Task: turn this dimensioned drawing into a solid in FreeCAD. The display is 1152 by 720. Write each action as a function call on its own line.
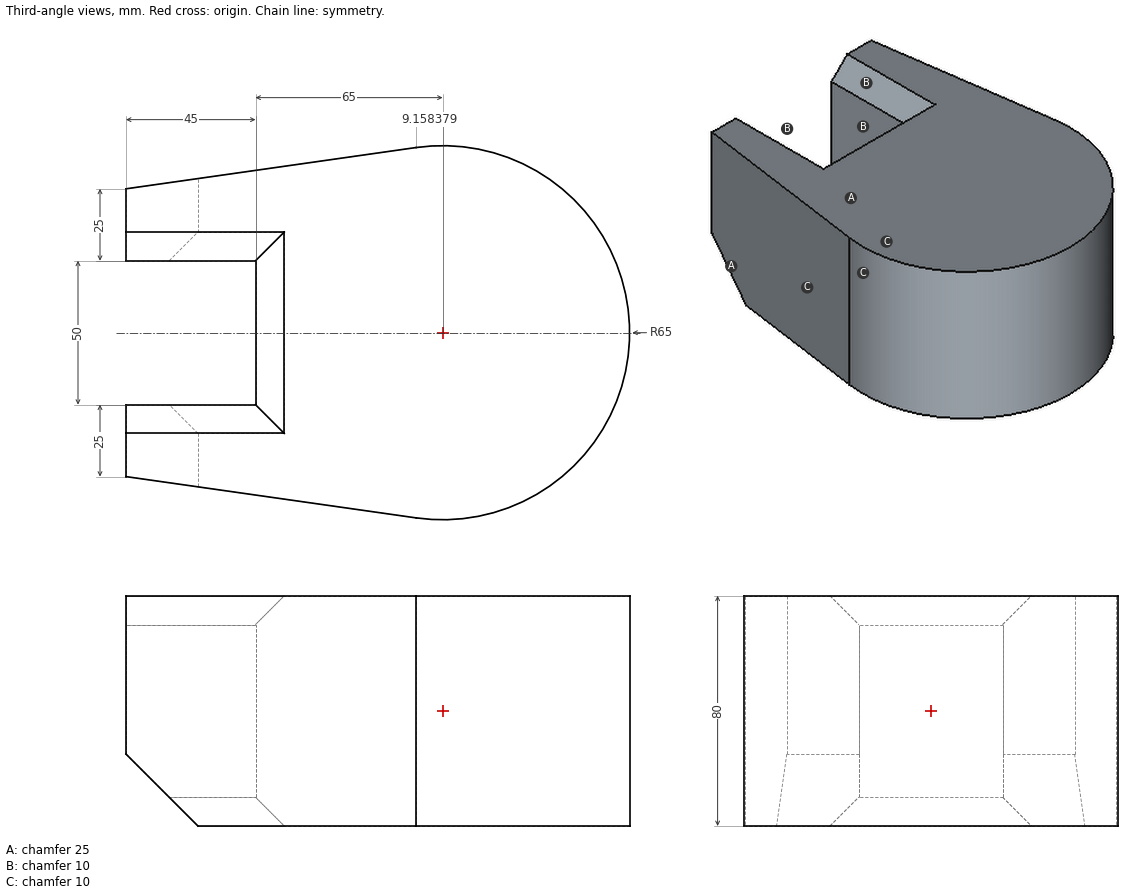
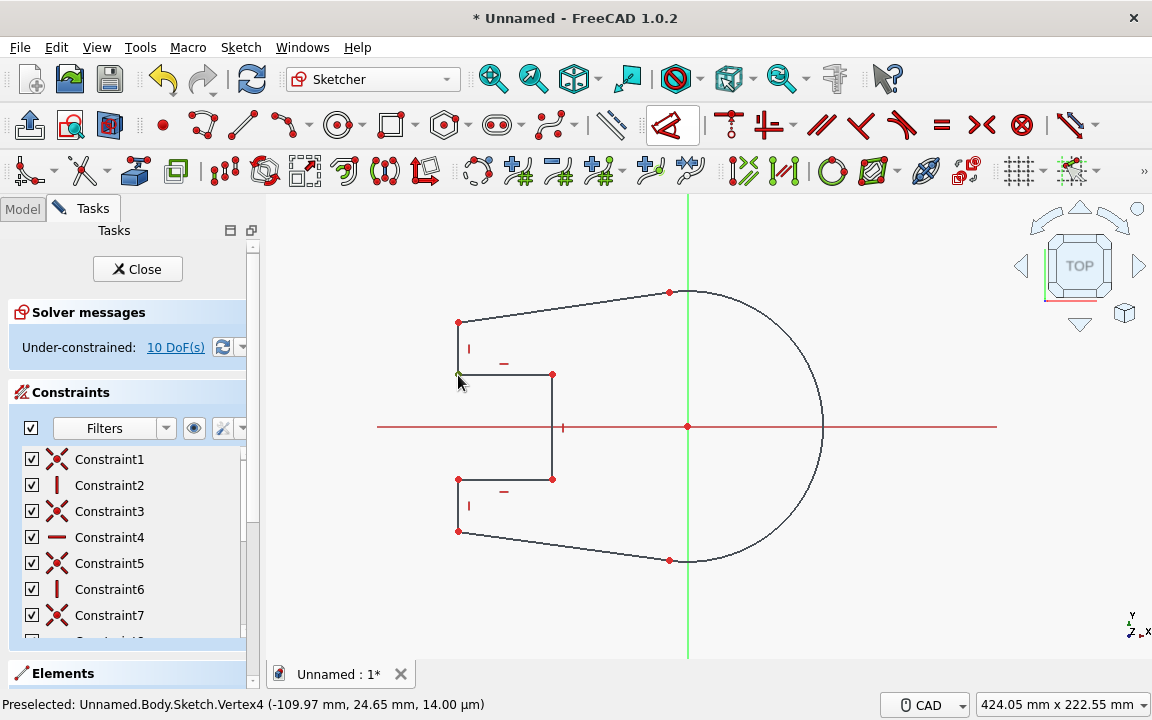
click(458, 480)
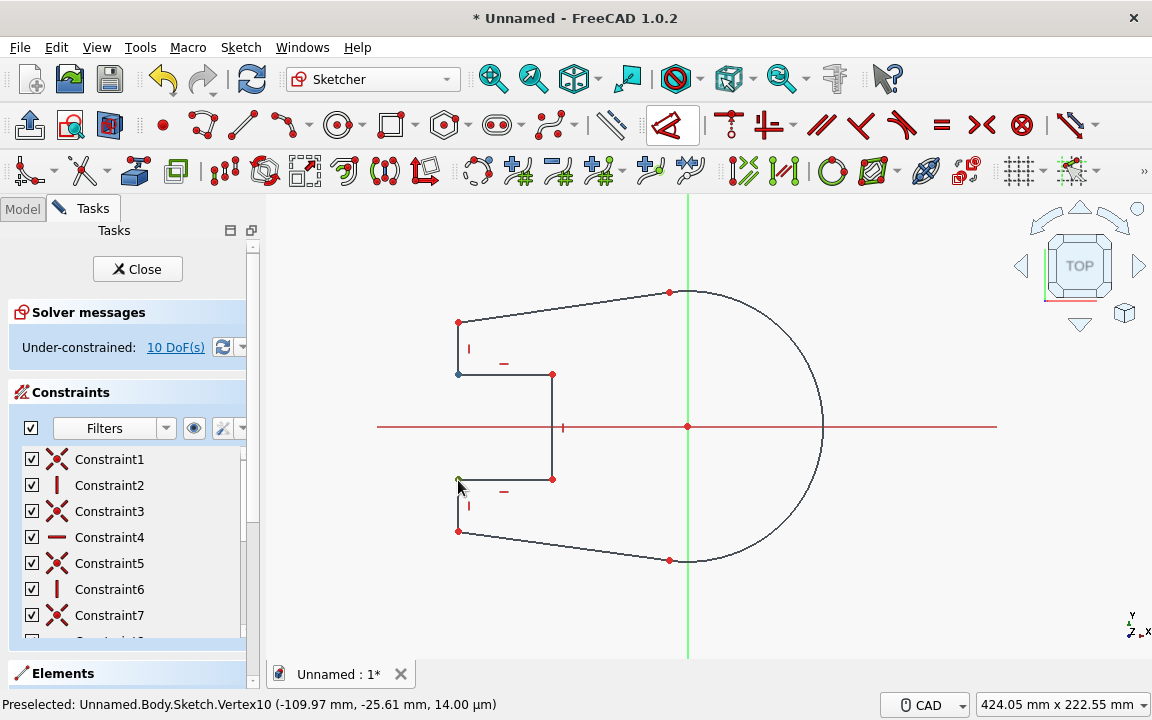
click(393, 426)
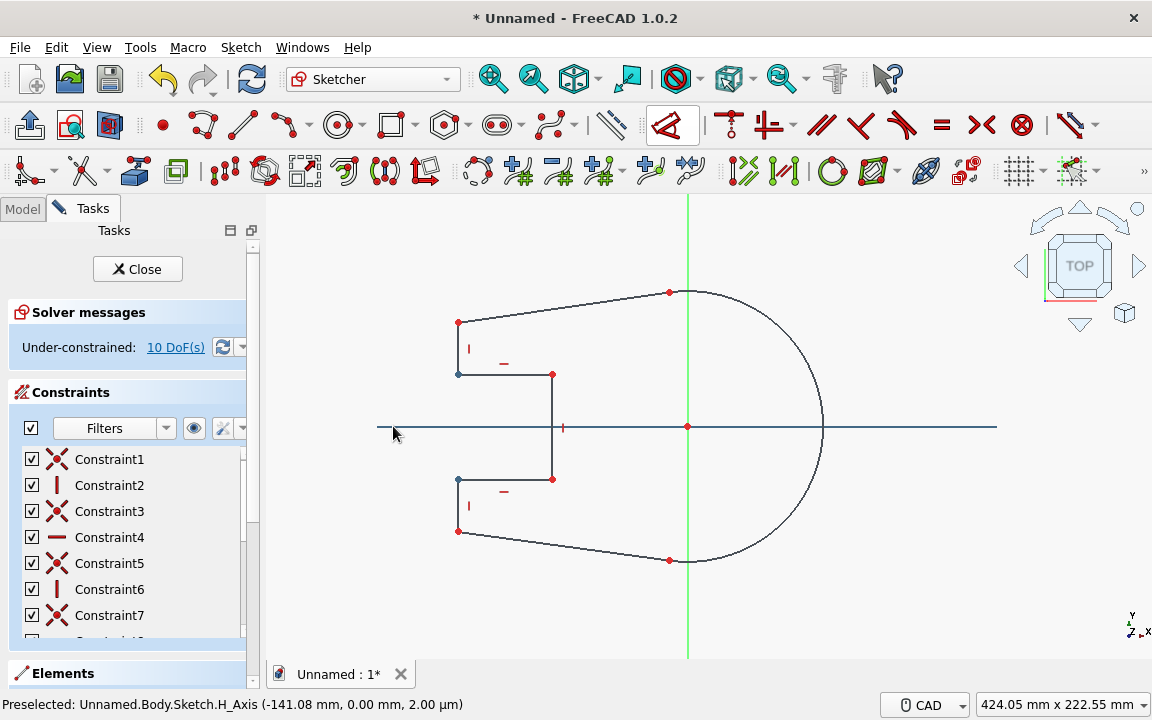
click(982, 126)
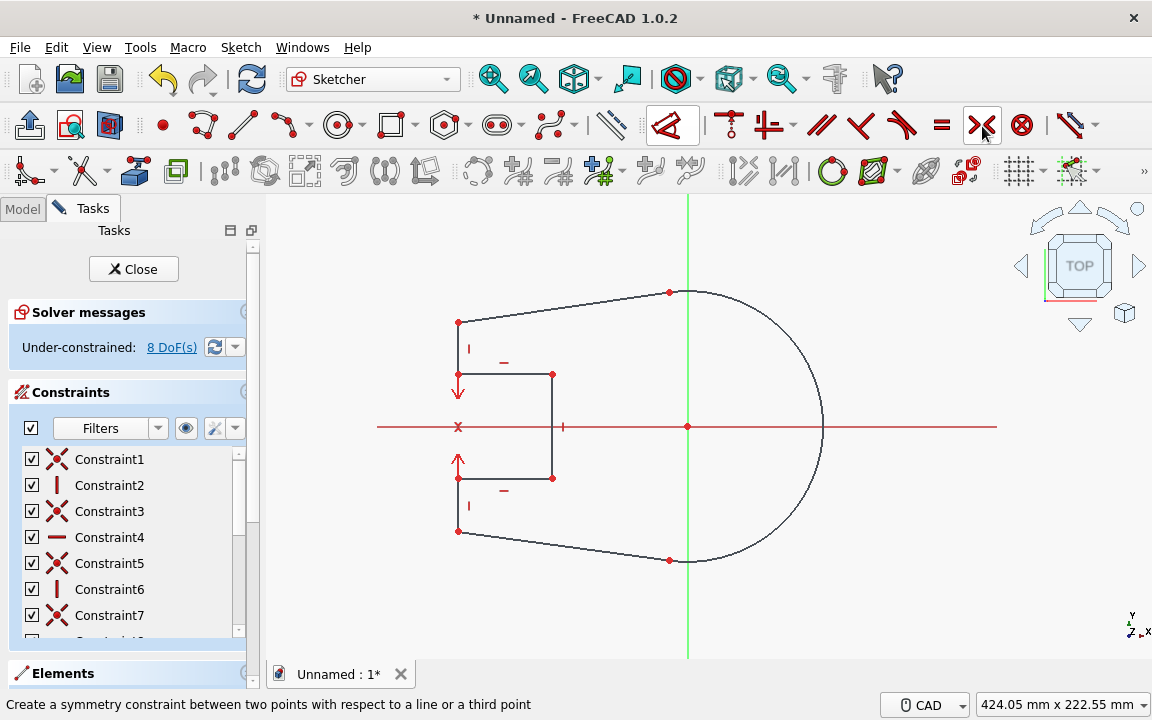
click(666, 126)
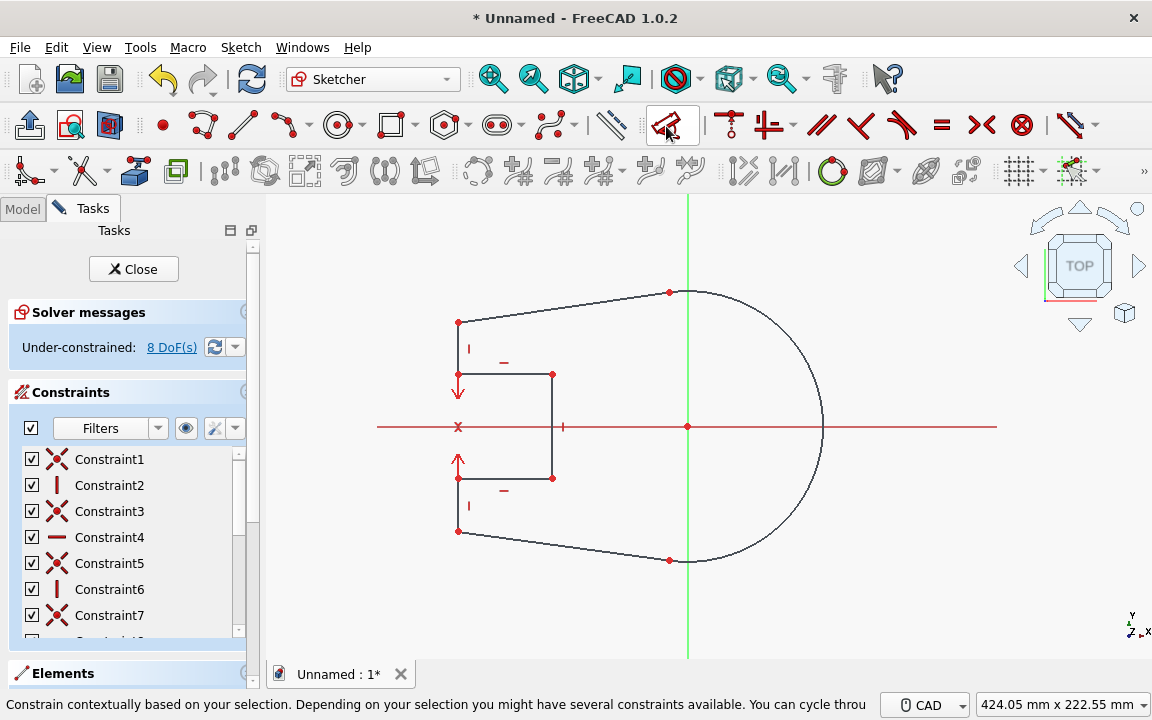
click(793, 512)
click(818, 532)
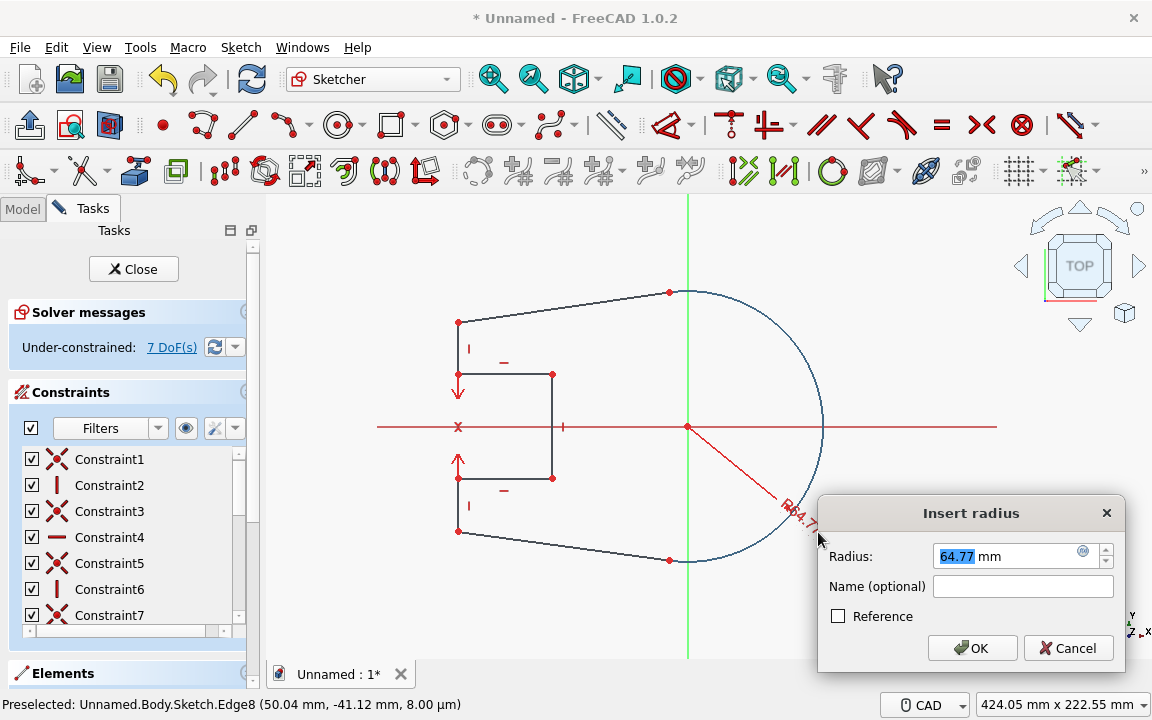
text(65)
key(Return)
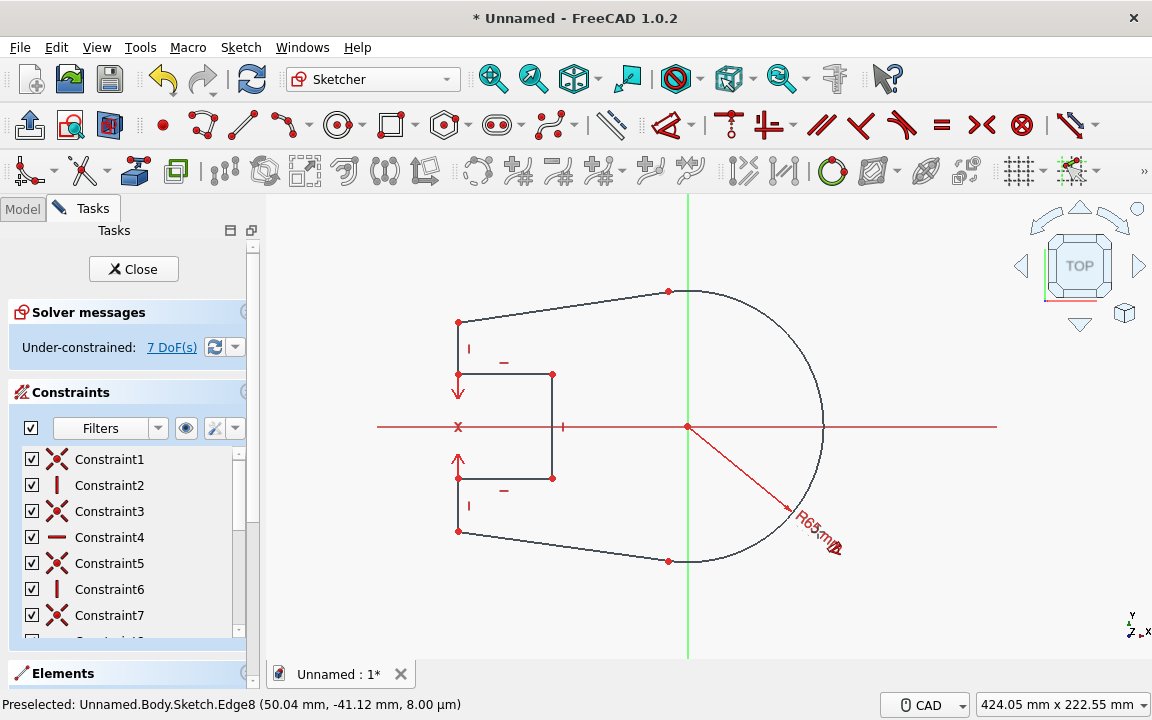
click(458, 338)
click(424, 349)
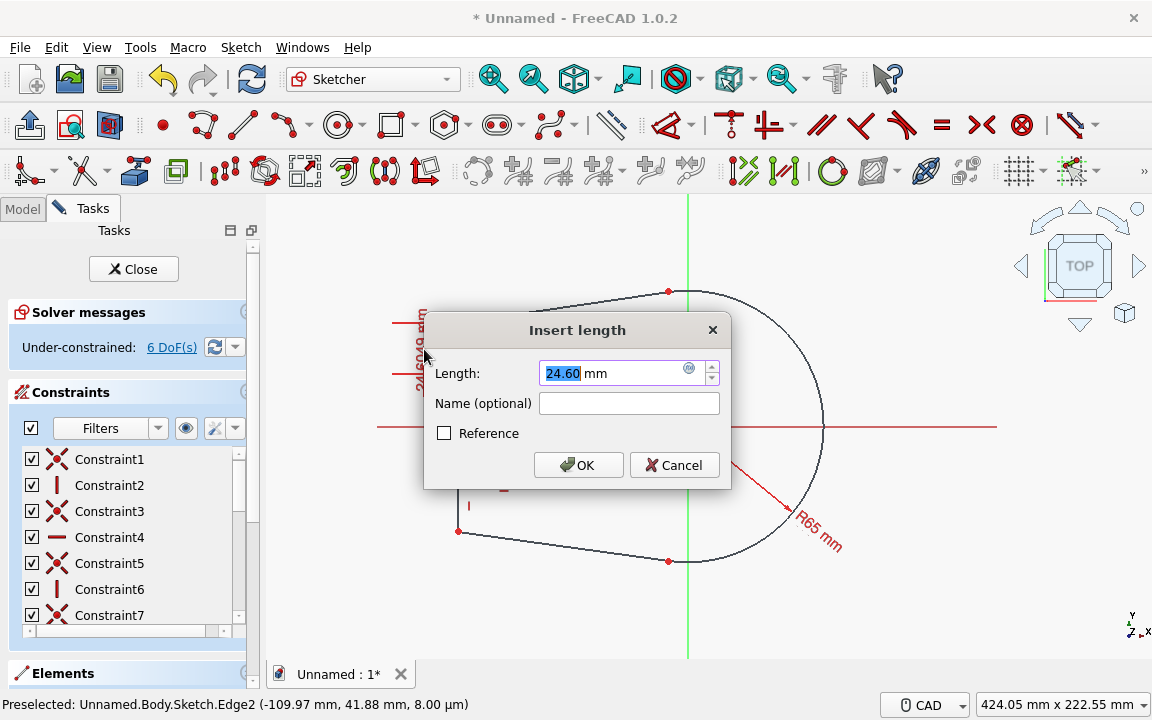
text(25)
key(Return)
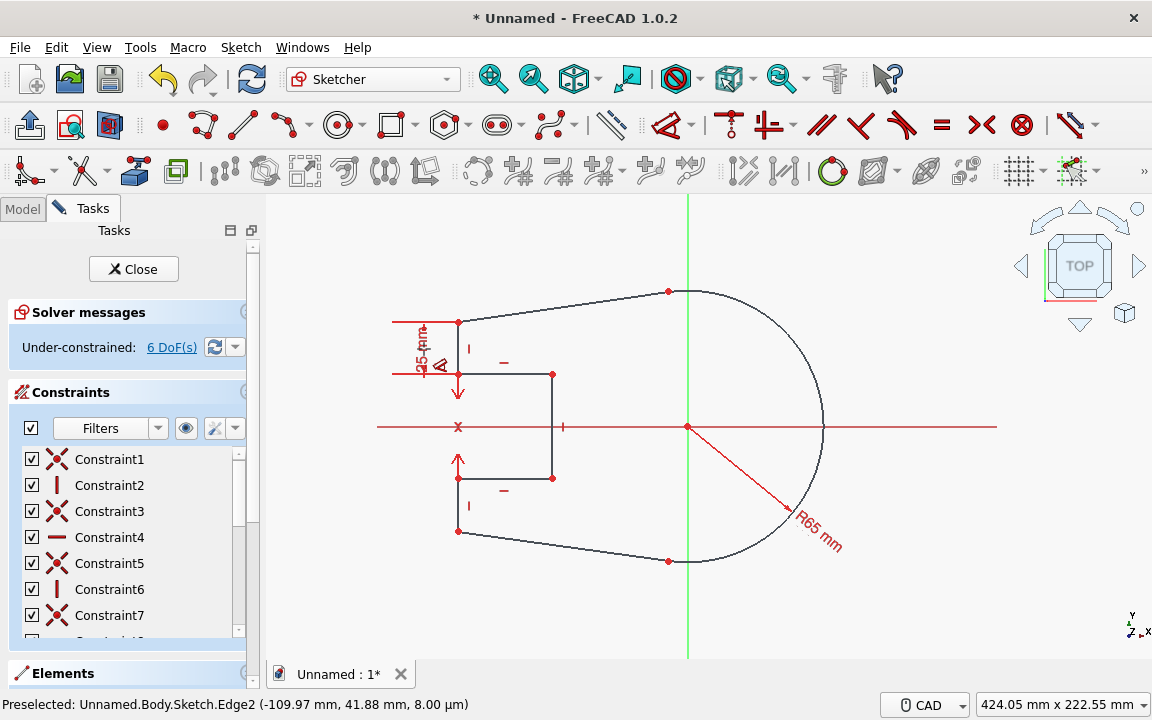
click(486, 374)
click(505, 340)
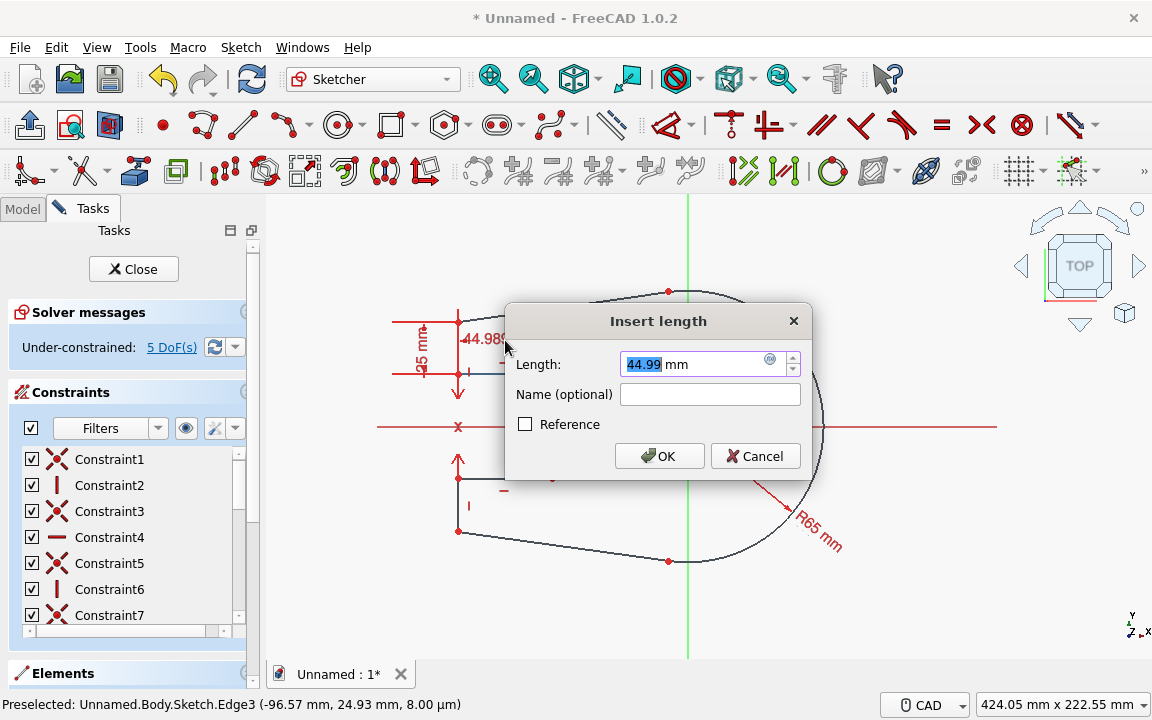
text(45)
key(Return)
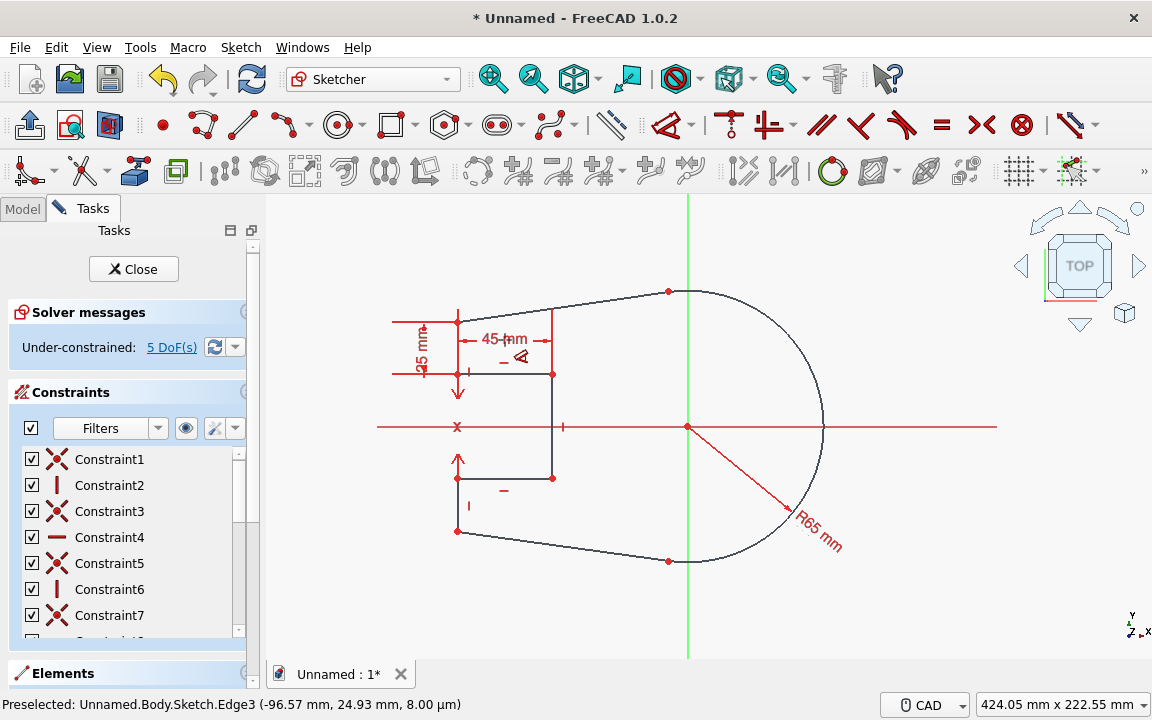
click(552, 406)
click(518, 403)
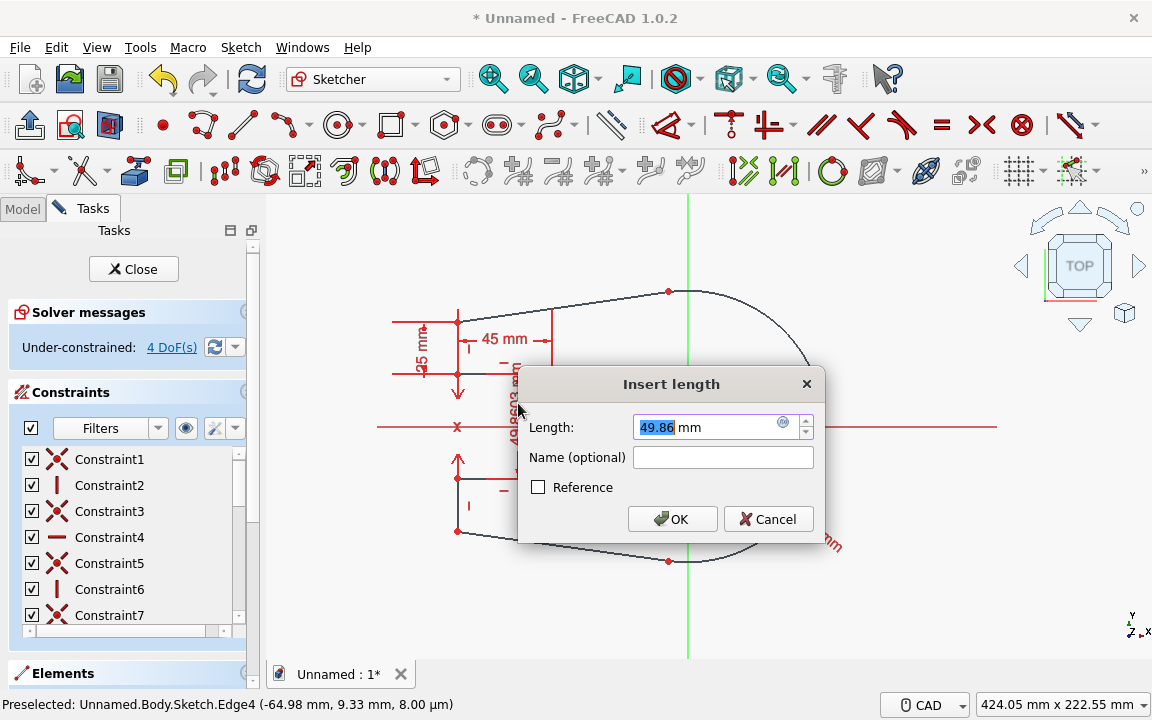
text(50)
key(Return)